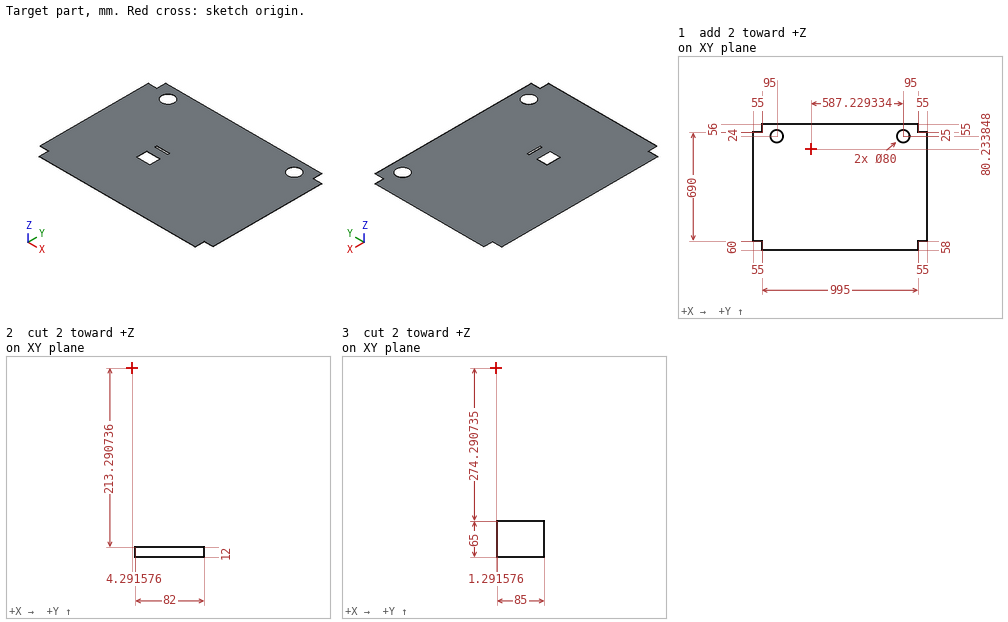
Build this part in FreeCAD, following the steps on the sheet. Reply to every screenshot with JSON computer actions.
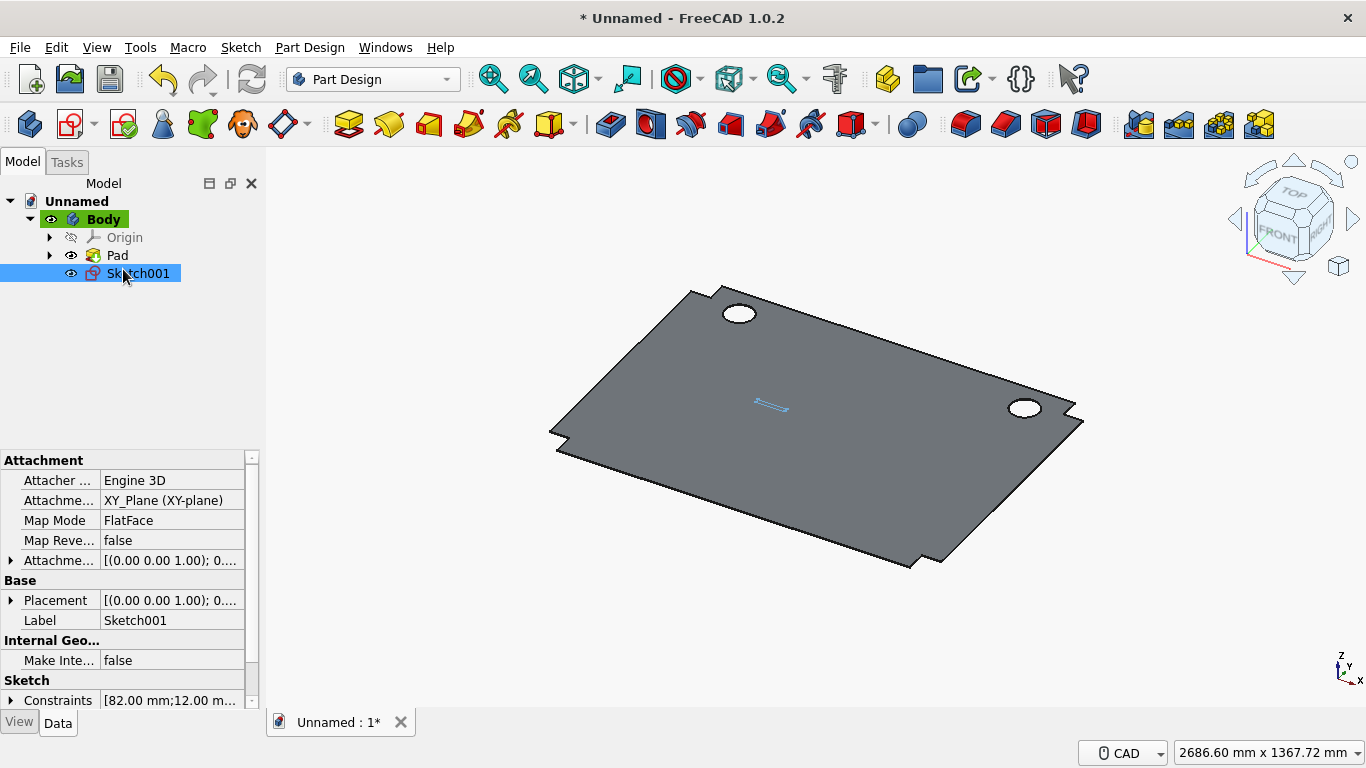
{"action": "left_click", "coordinate": [612, 124]}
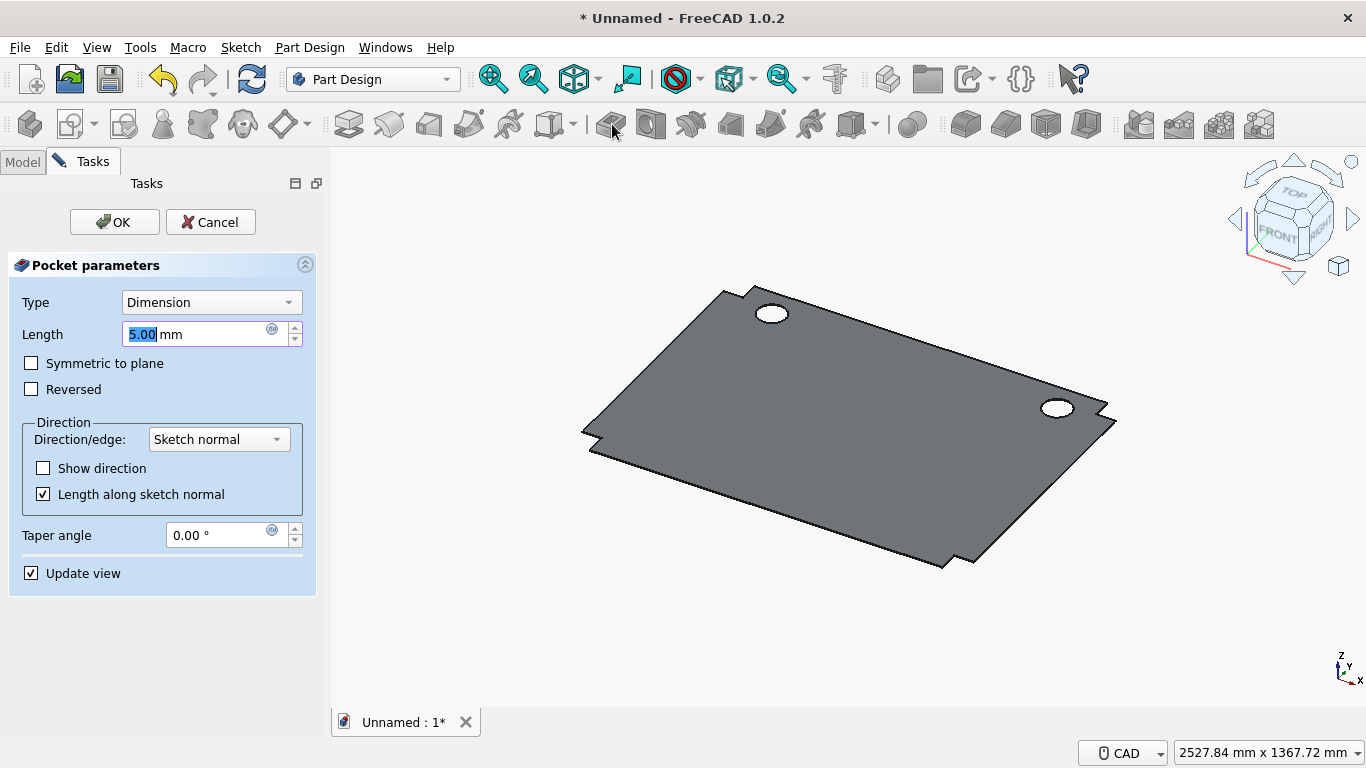
{"action": "type", "text": "2"}
{"action": "key", "text": "Tab"}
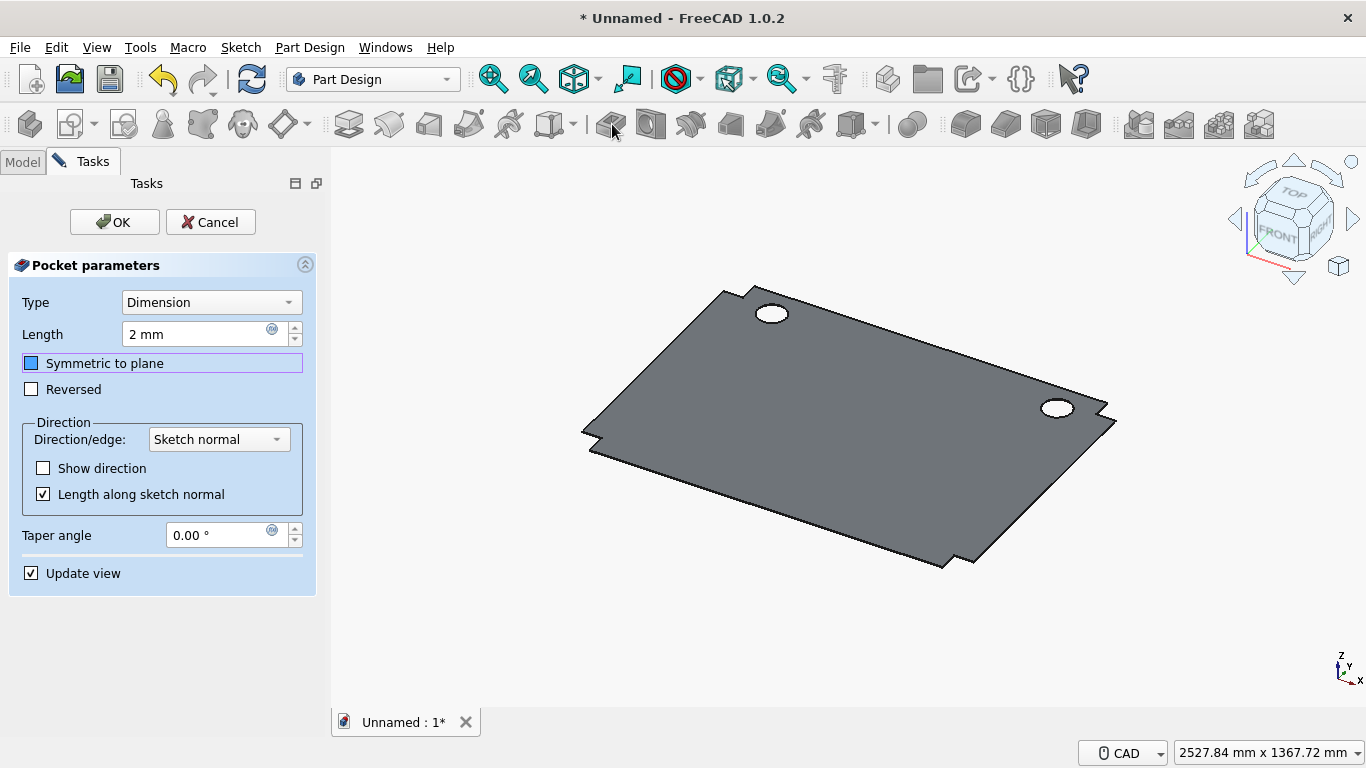
{"action": "left_click", "coordinate": [30, 389]}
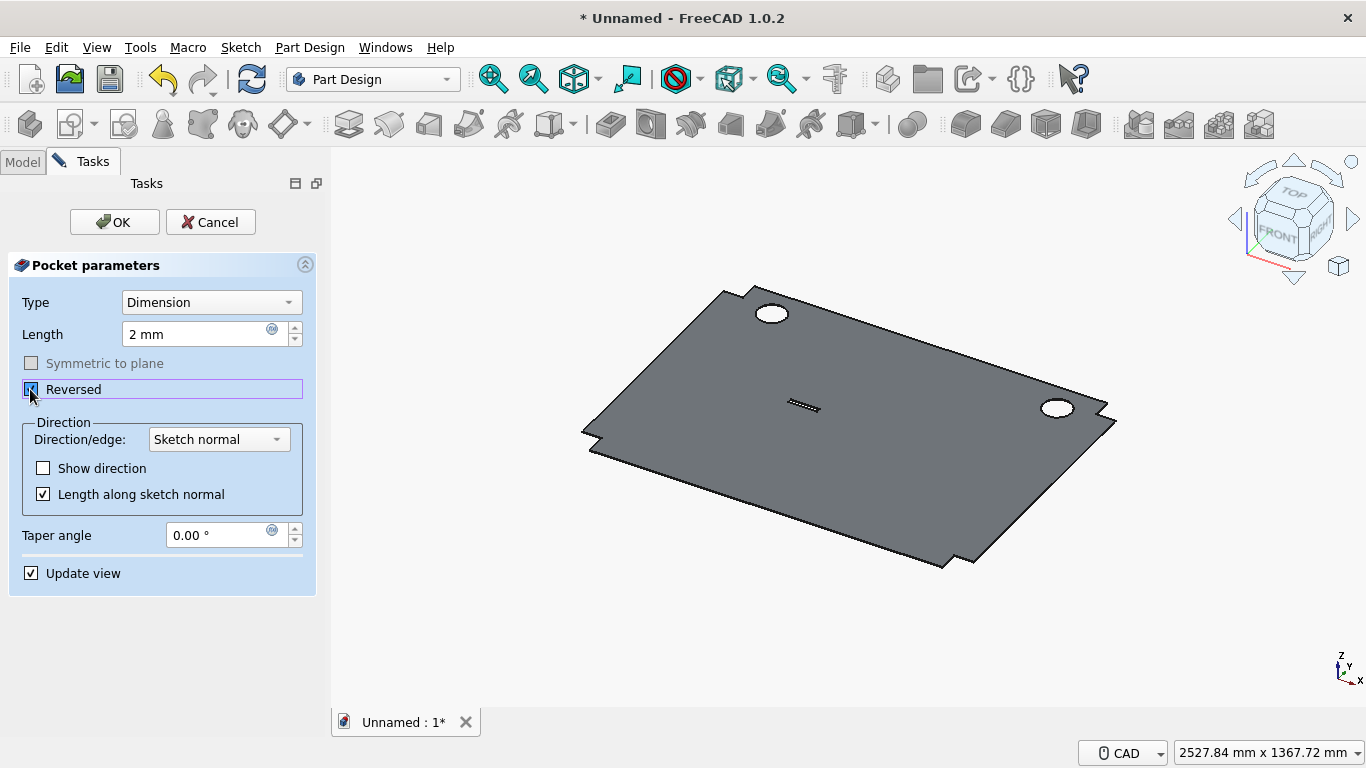
{"action": "left_click", "coordinate": [115, 222]}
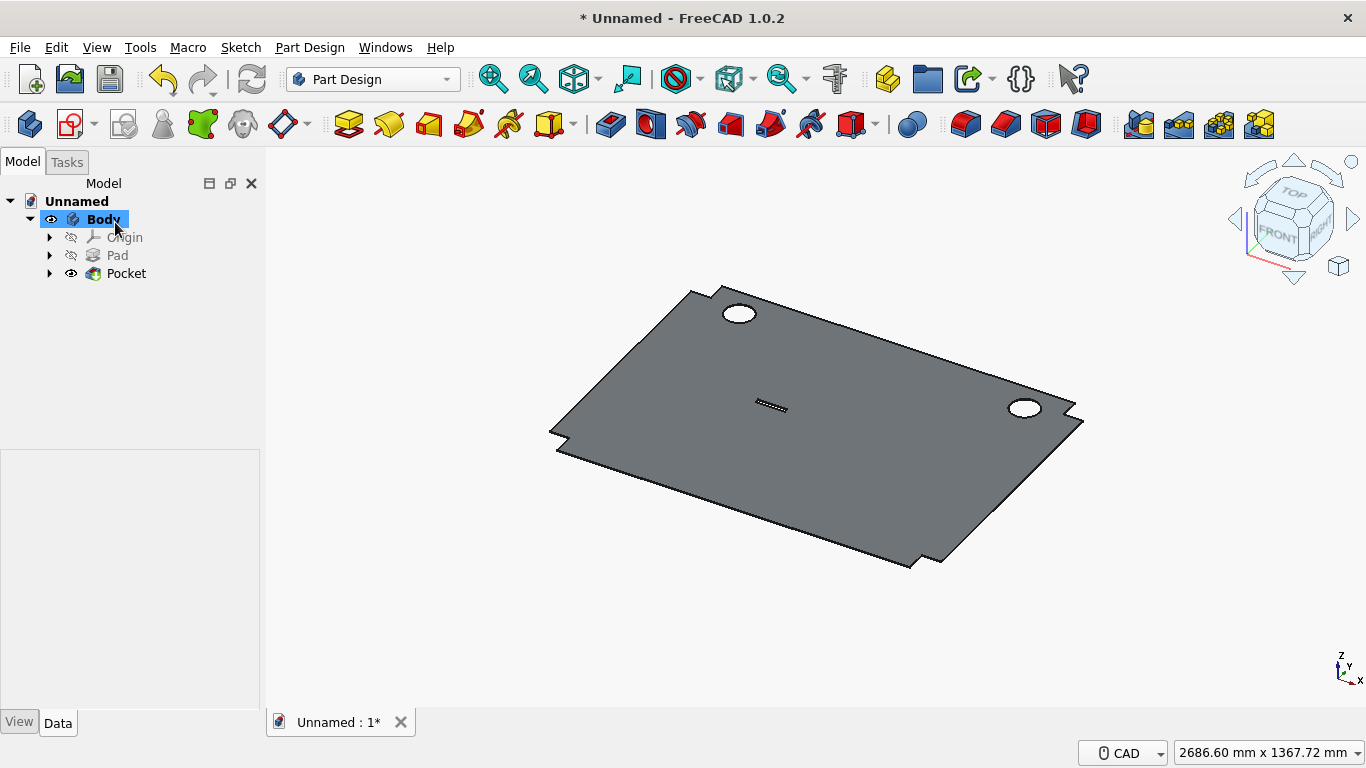
{"action": "left_click", "coordinate": [70, 124]}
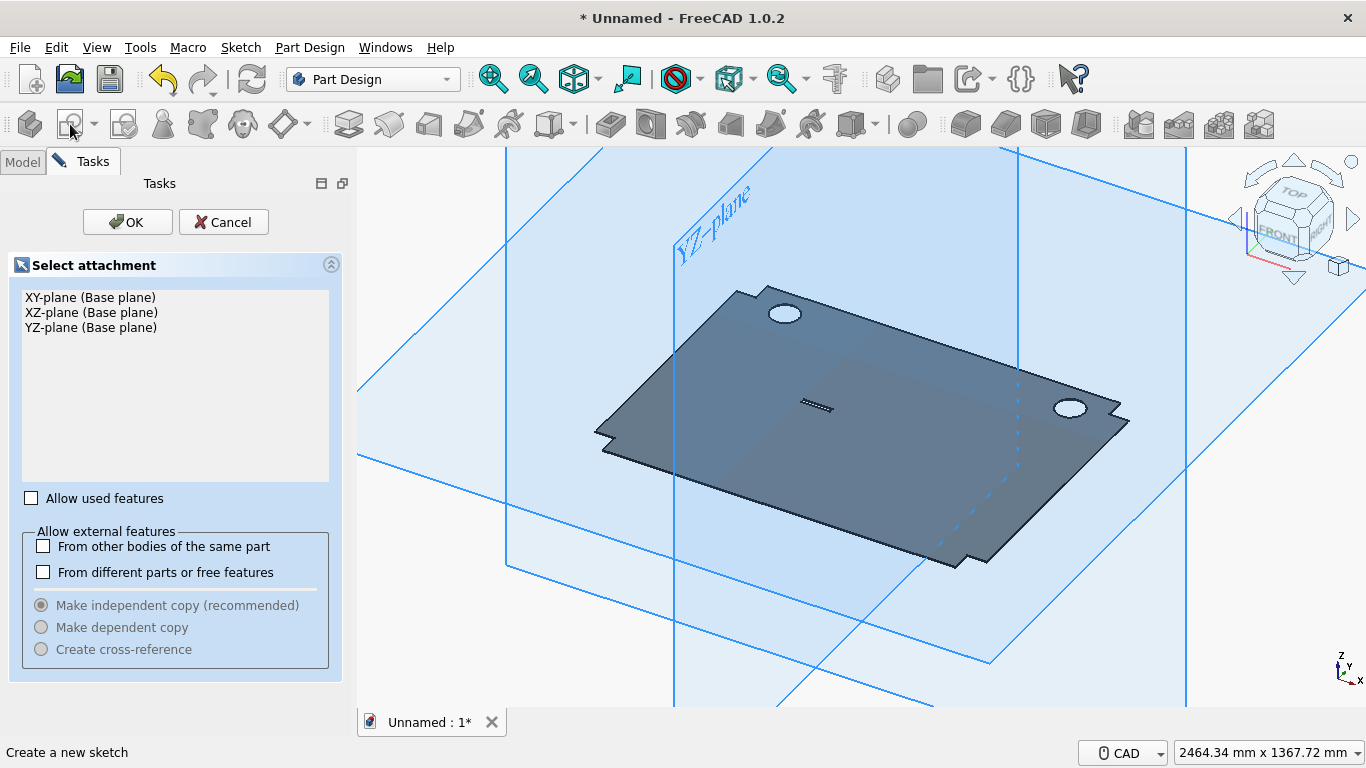
{"action": "left_click", "coordinate": [82, 298]}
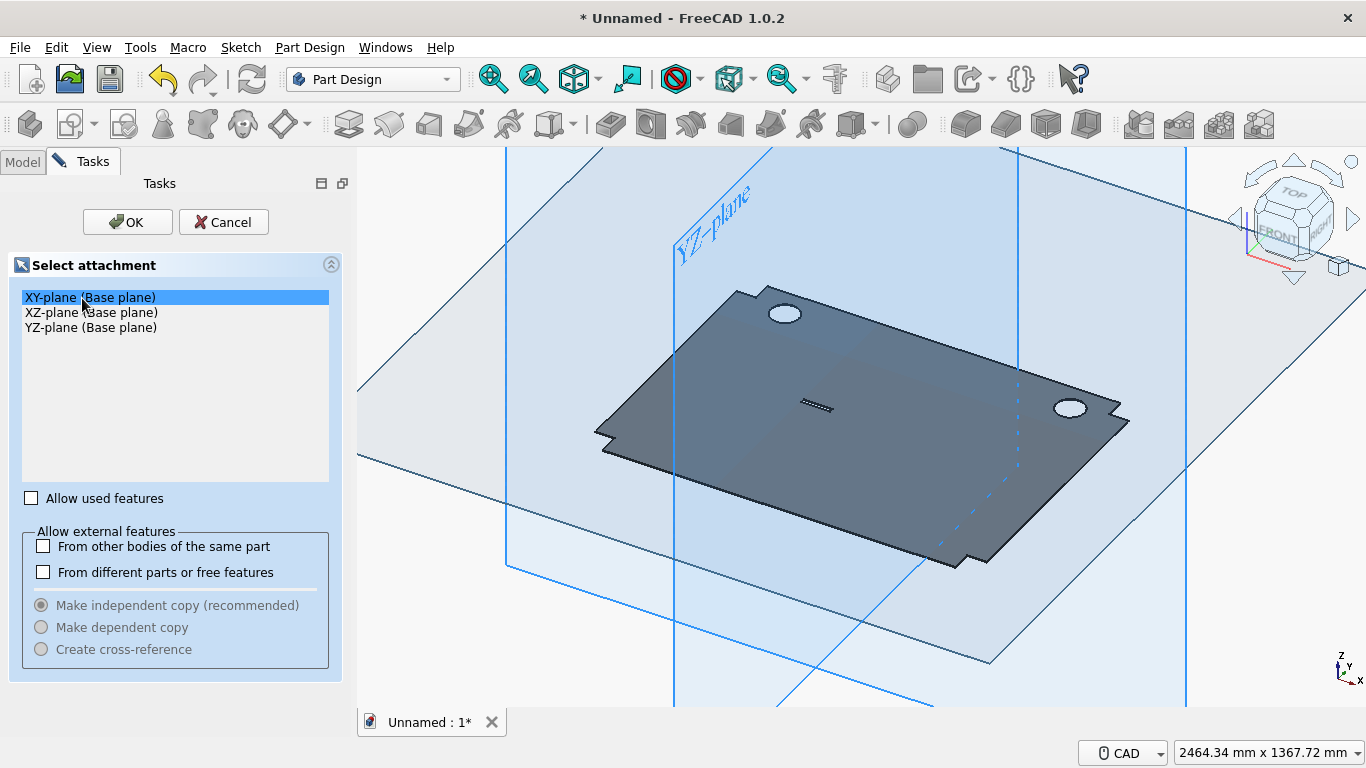
{"action": "left_click", "coordinate": [128, 222]}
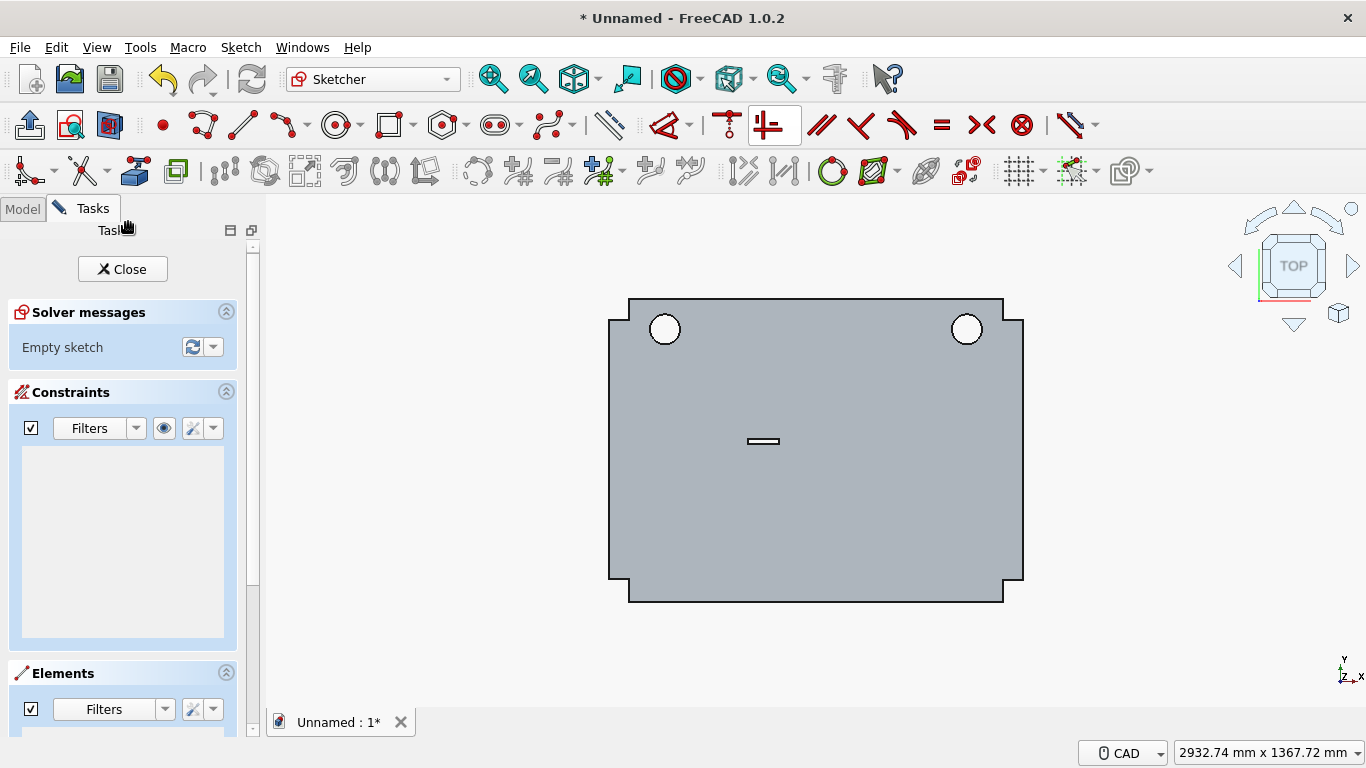
{"action": "left_click", "coordinate": [110, 126]}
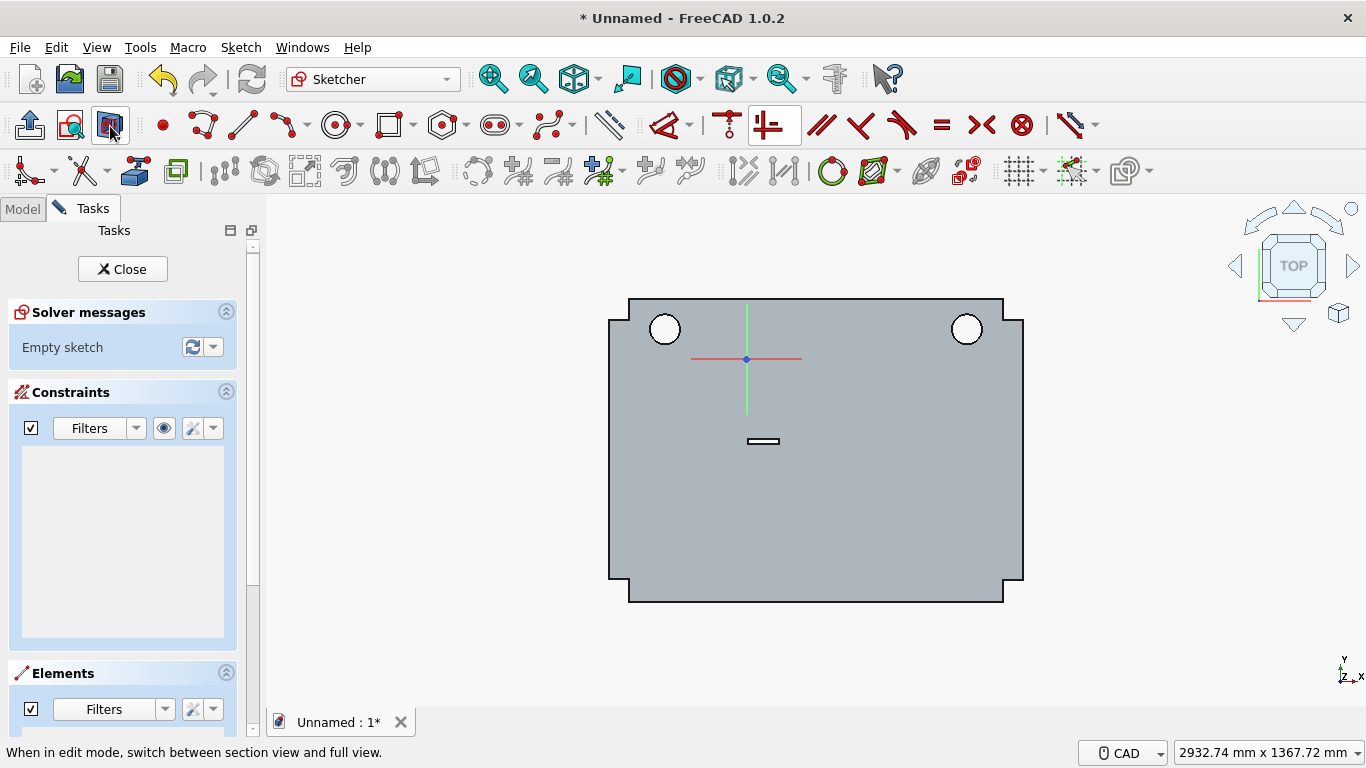
{"action": "scroll", "coordinate": [764, 476], "scroll_direction": "up", "scroll_amount": 13}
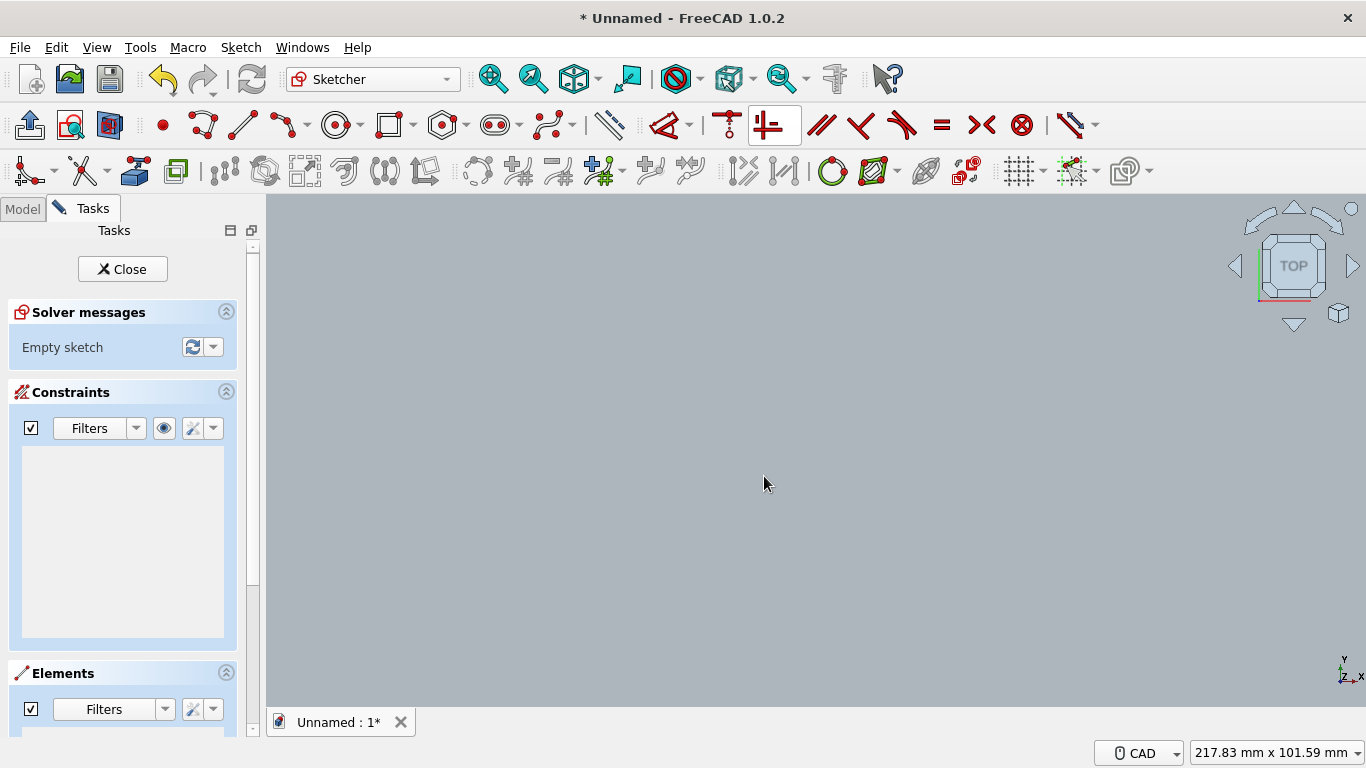
{"action": "left_click", "coordinate": [390, 126]}